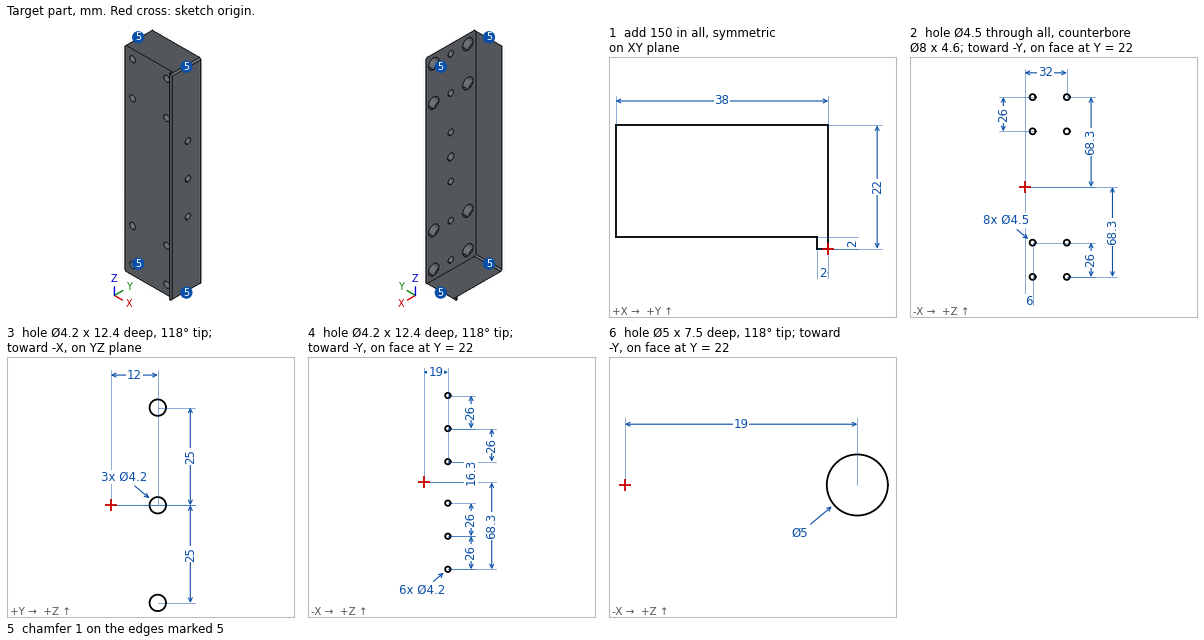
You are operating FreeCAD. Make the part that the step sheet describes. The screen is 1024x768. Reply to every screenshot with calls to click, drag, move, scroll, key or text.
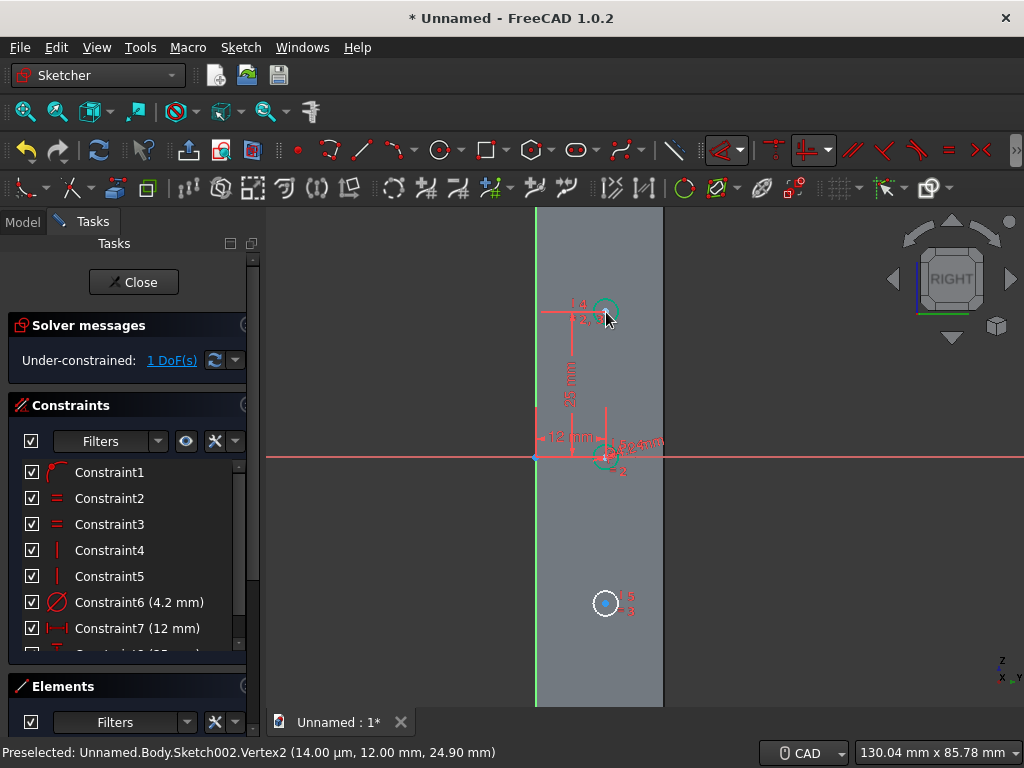
click(606, 604)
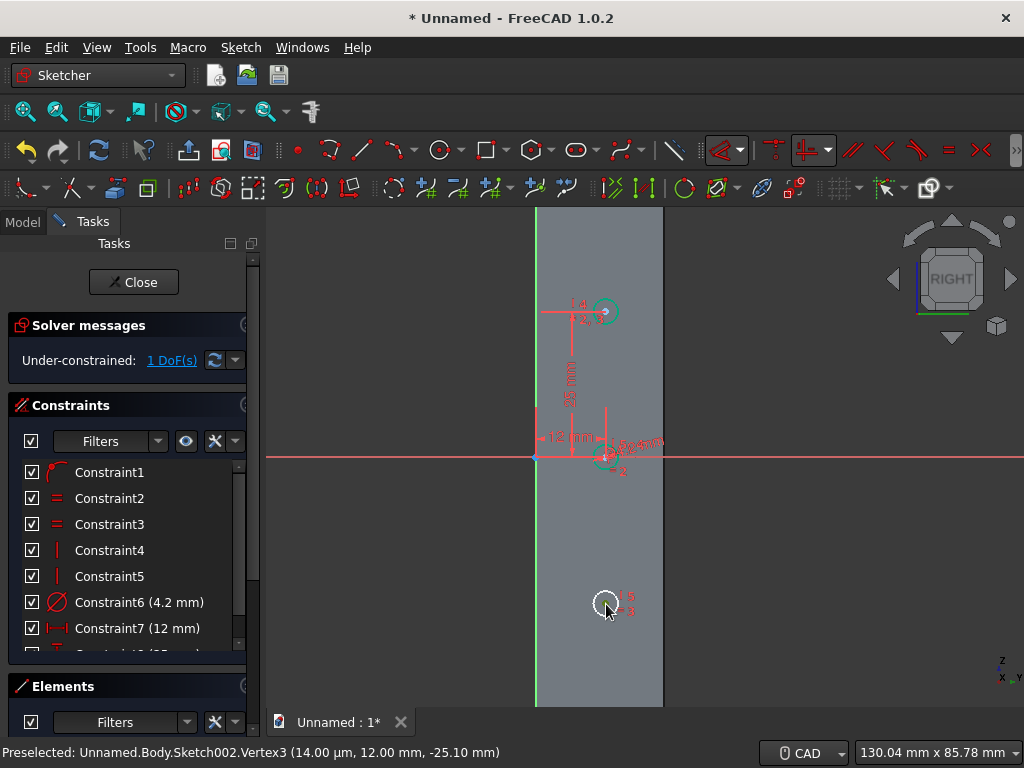
key(i)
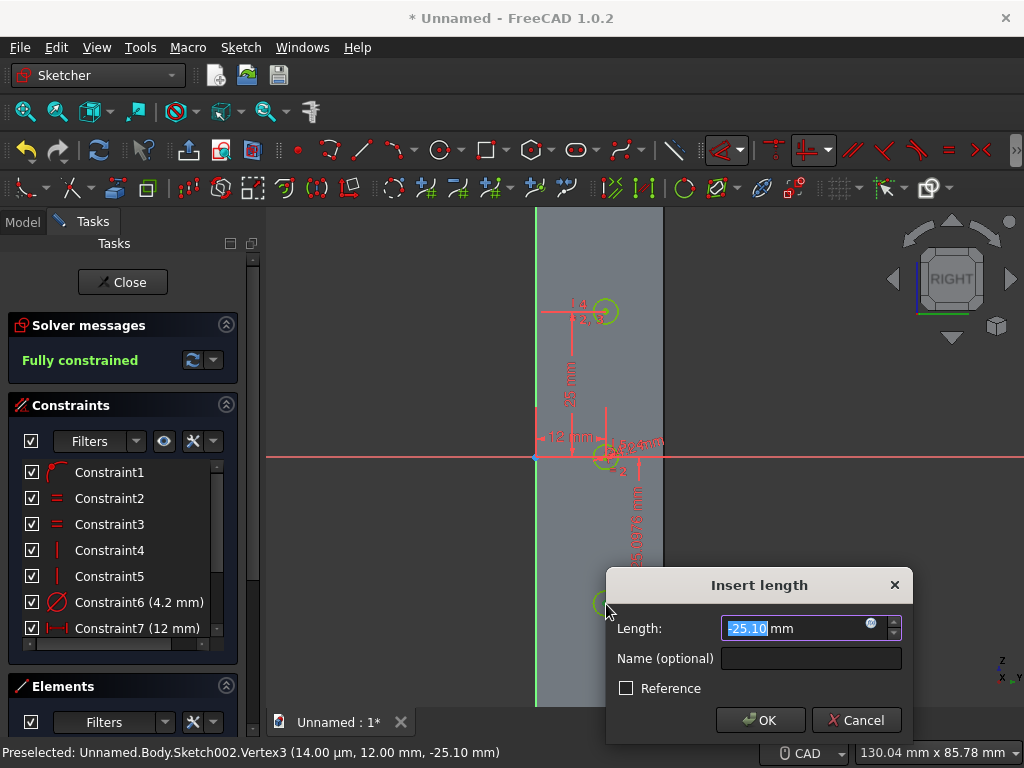
text(-25)
key(Return)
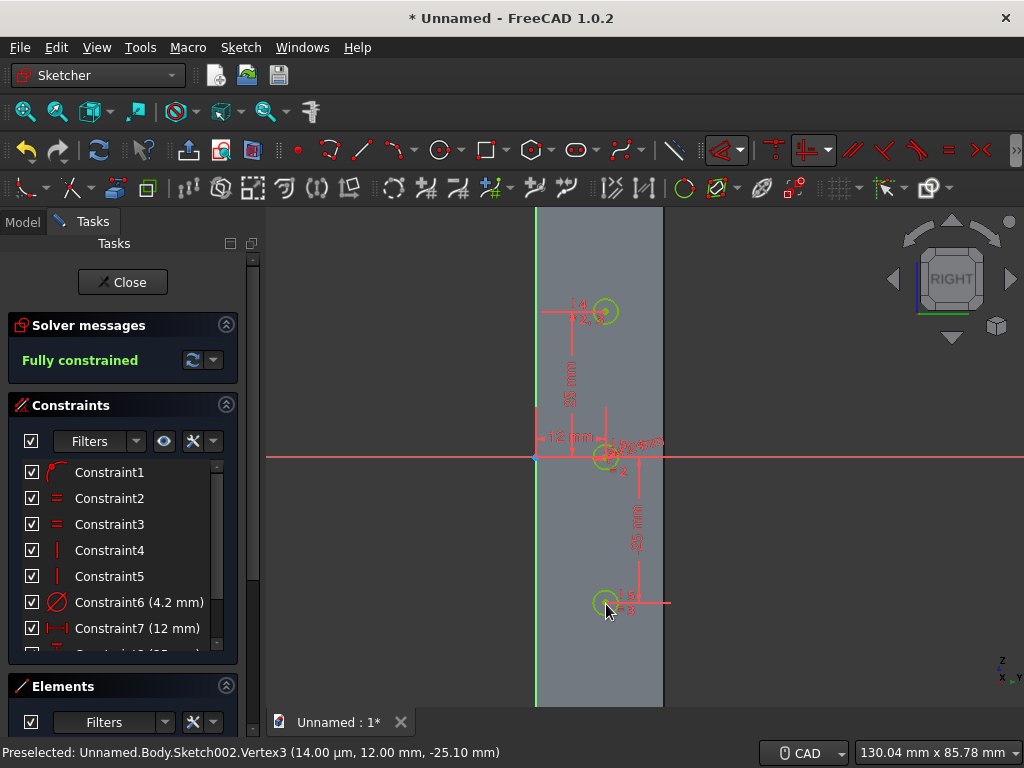
click(123, 282)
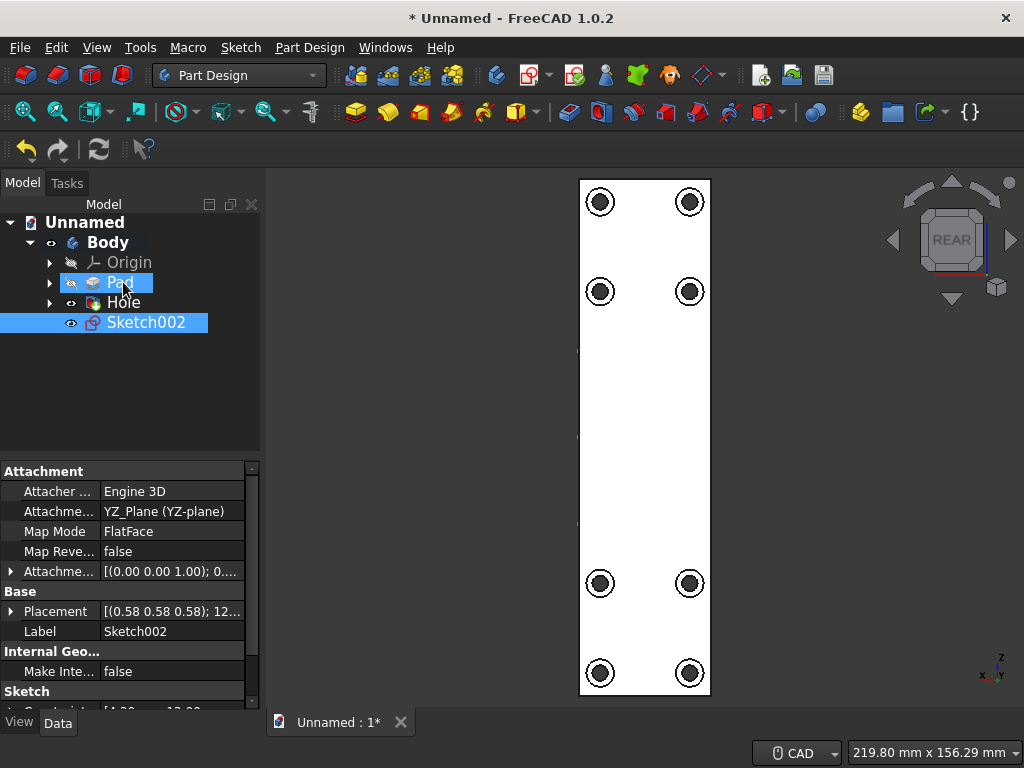
click(602, 112)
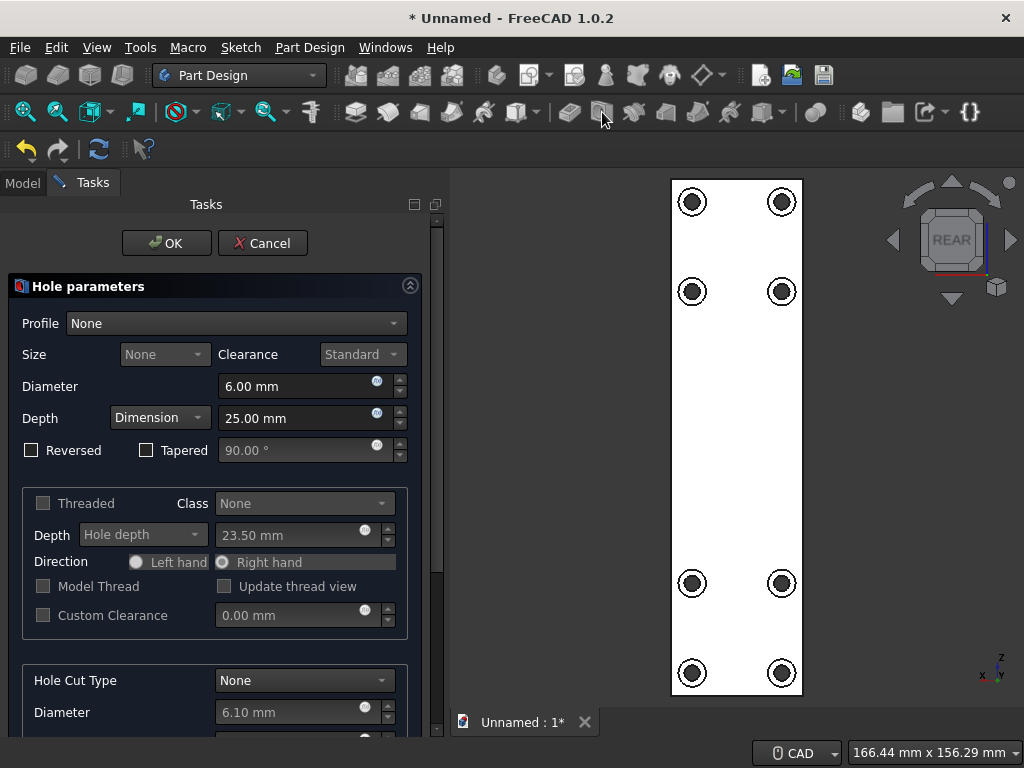
triple_click(305, 386)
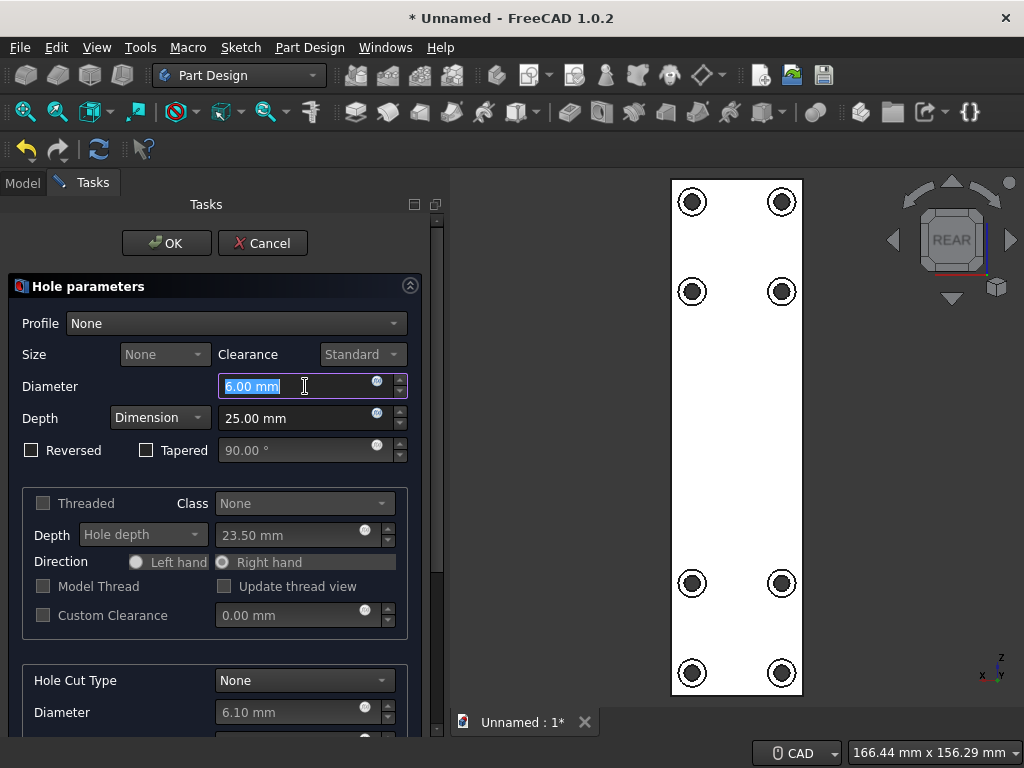
text(4.2)
key(Tab)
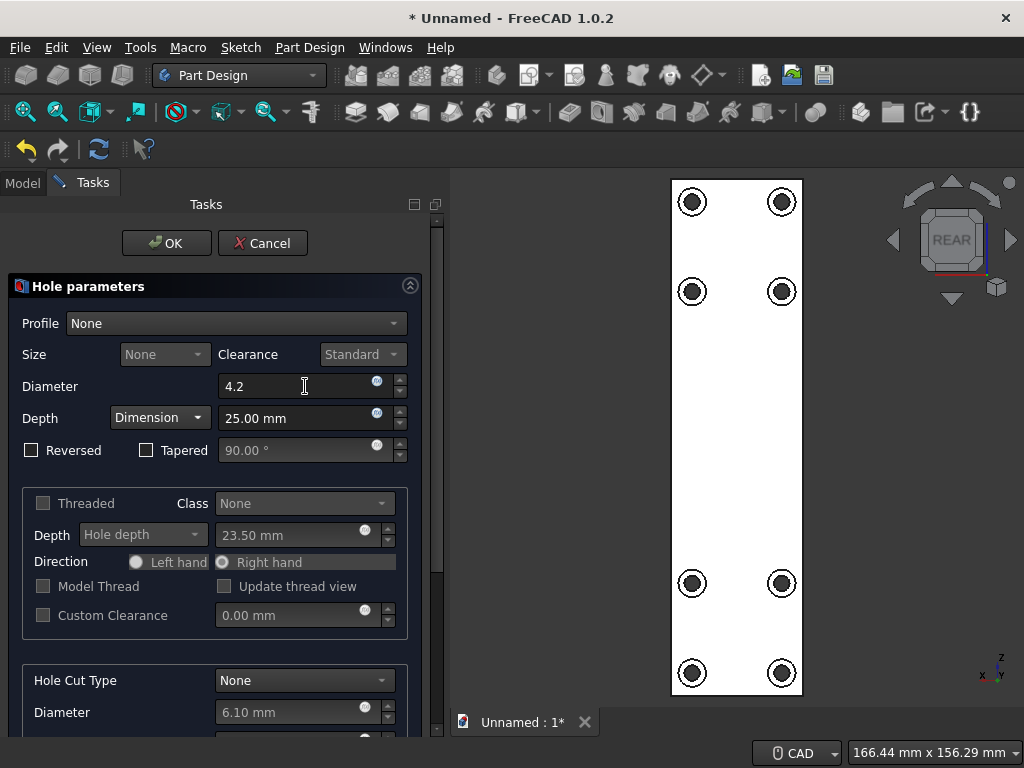
triple_click(305, 418)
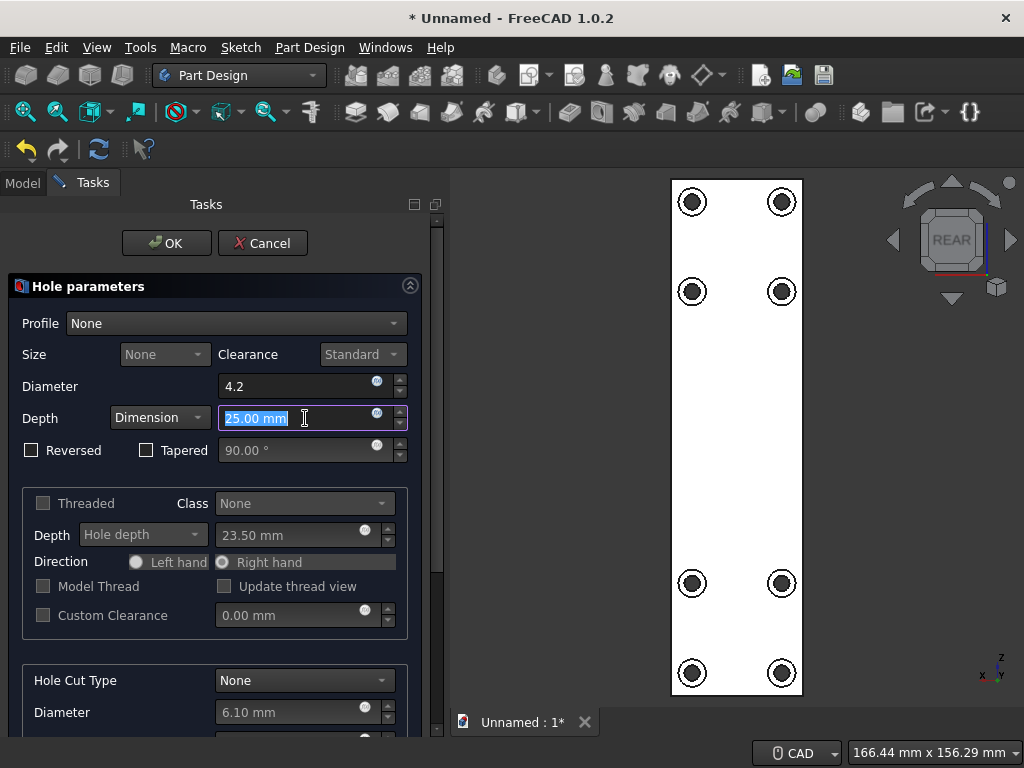
text(12.4)
key(Tab)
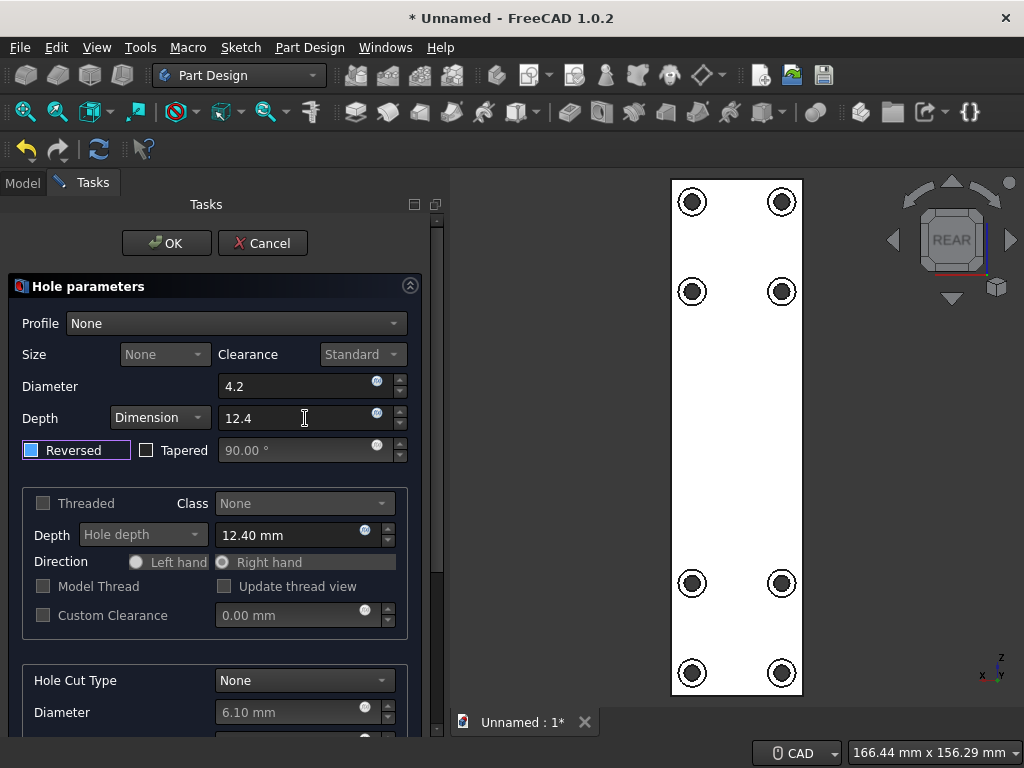
click(167, 243)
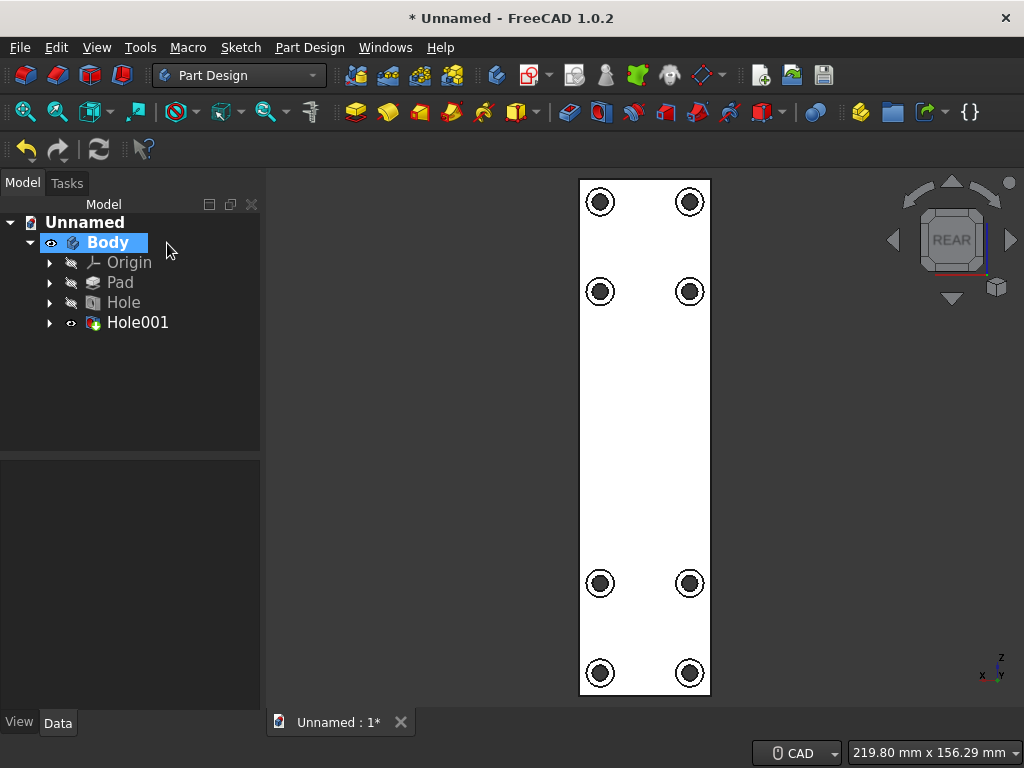
click(645, 363)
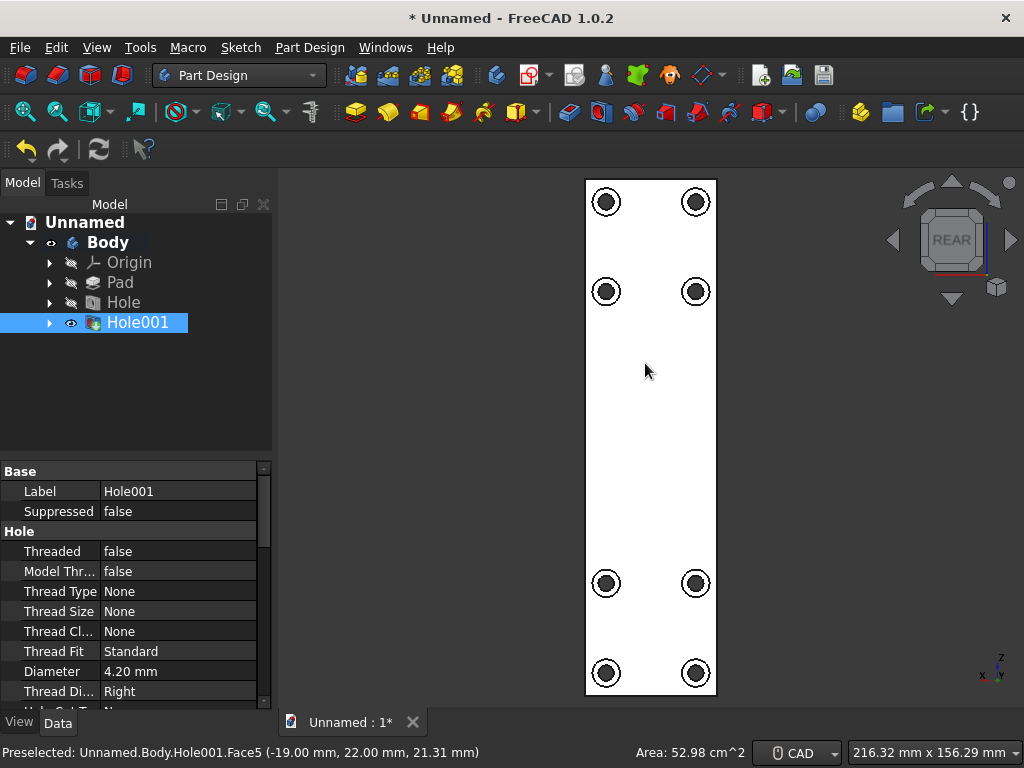
click(530, 76)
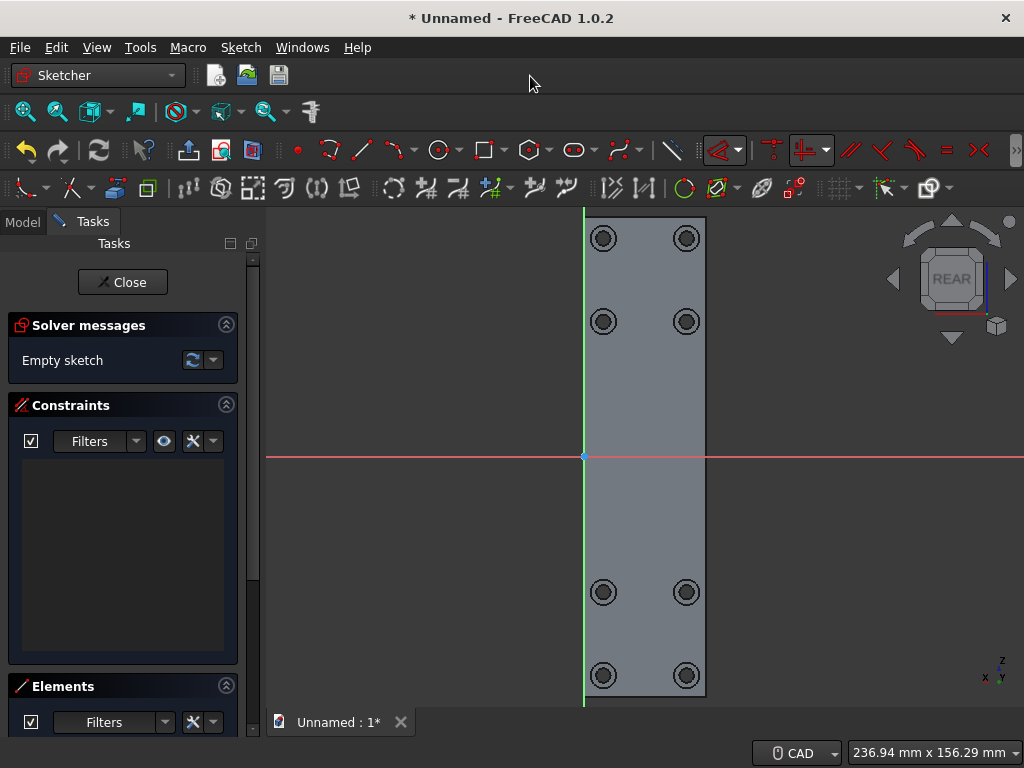
scroll(492, 457, down, 2)